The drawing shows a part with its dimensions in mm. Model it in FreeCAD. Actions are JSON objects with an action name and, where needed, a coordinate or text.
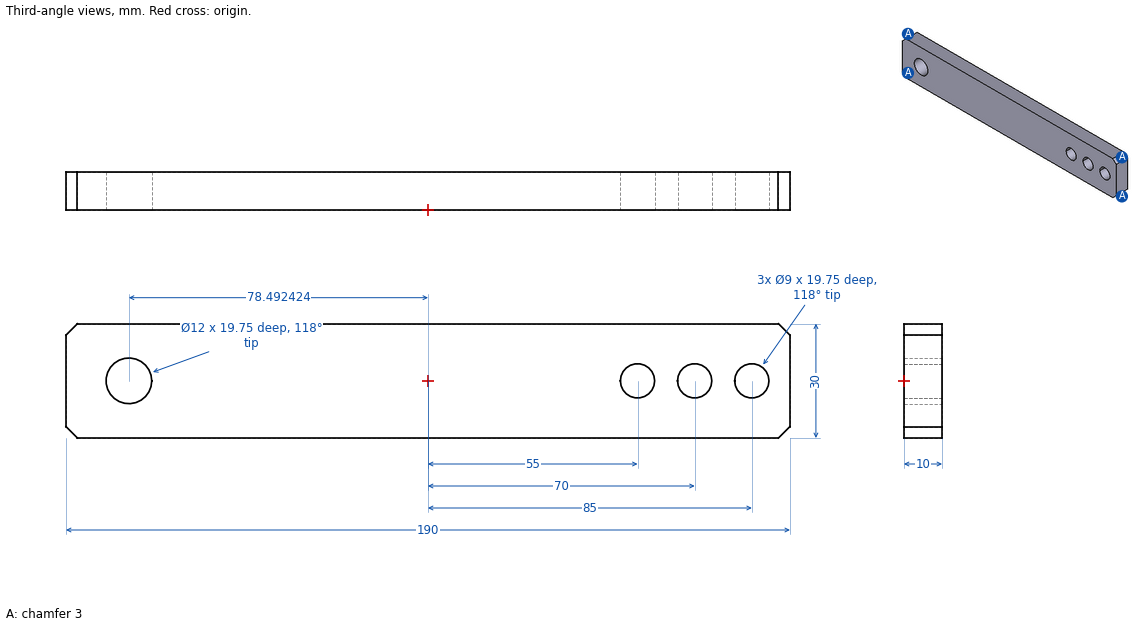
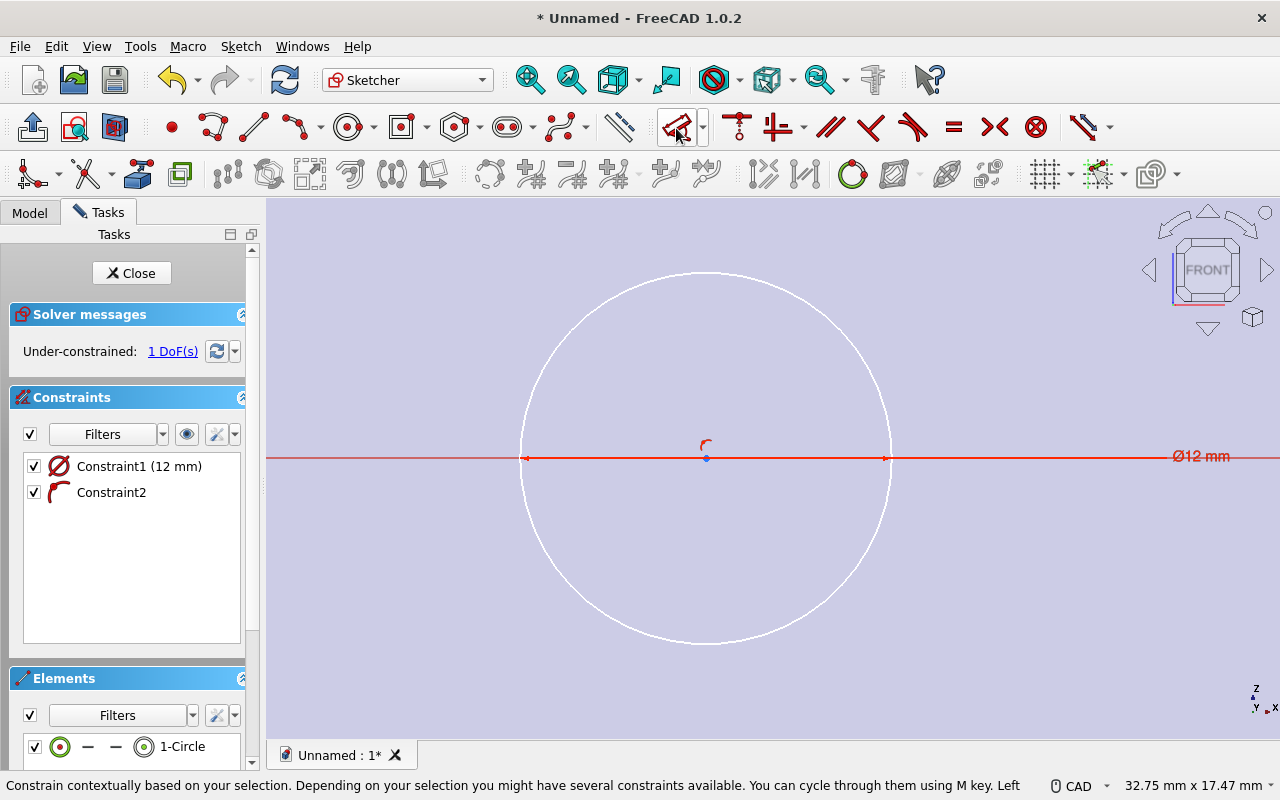
{"action": "left_click", "coordinate": [706, 458]}
{"action": "left_click", "coordinate": [911, 492]}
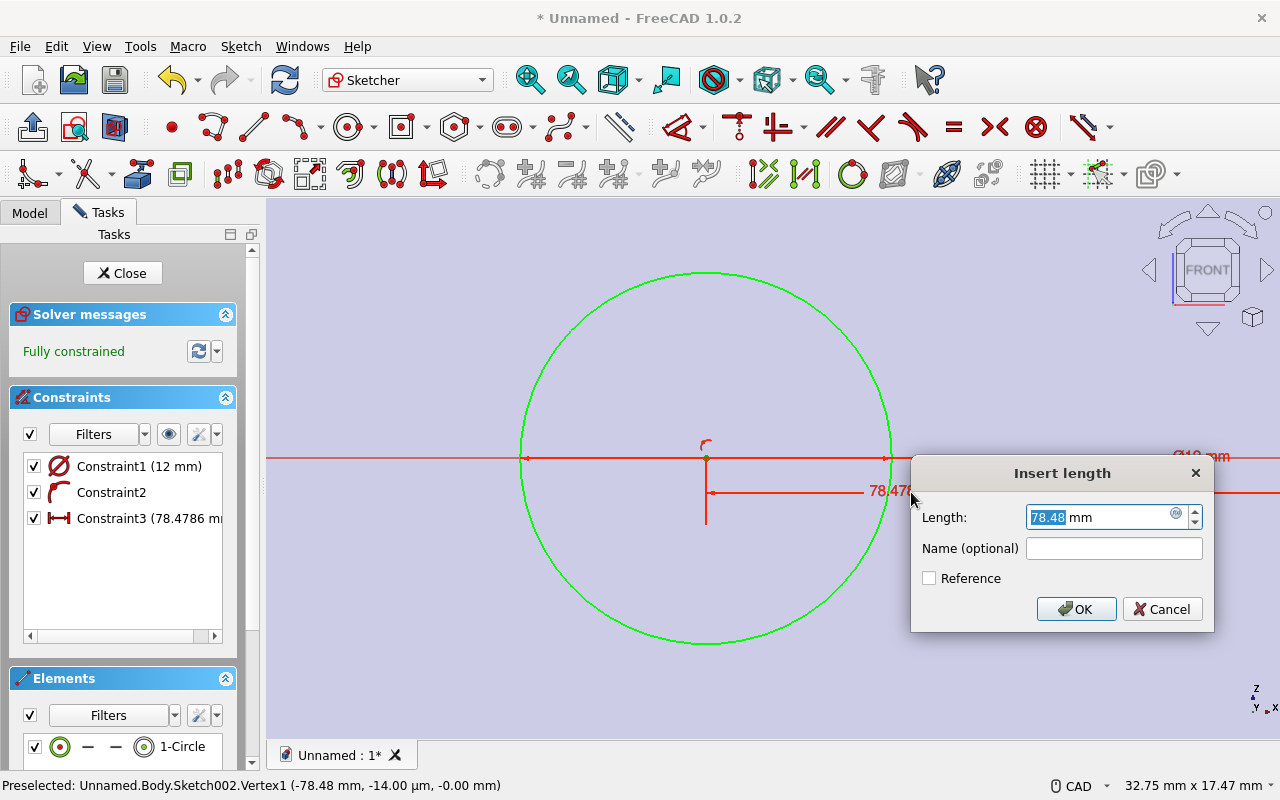
{"action": "type", "text": "78.492424"}
{"action": "key", "text": "Return"}
{"action": "key", "text": "Escape"}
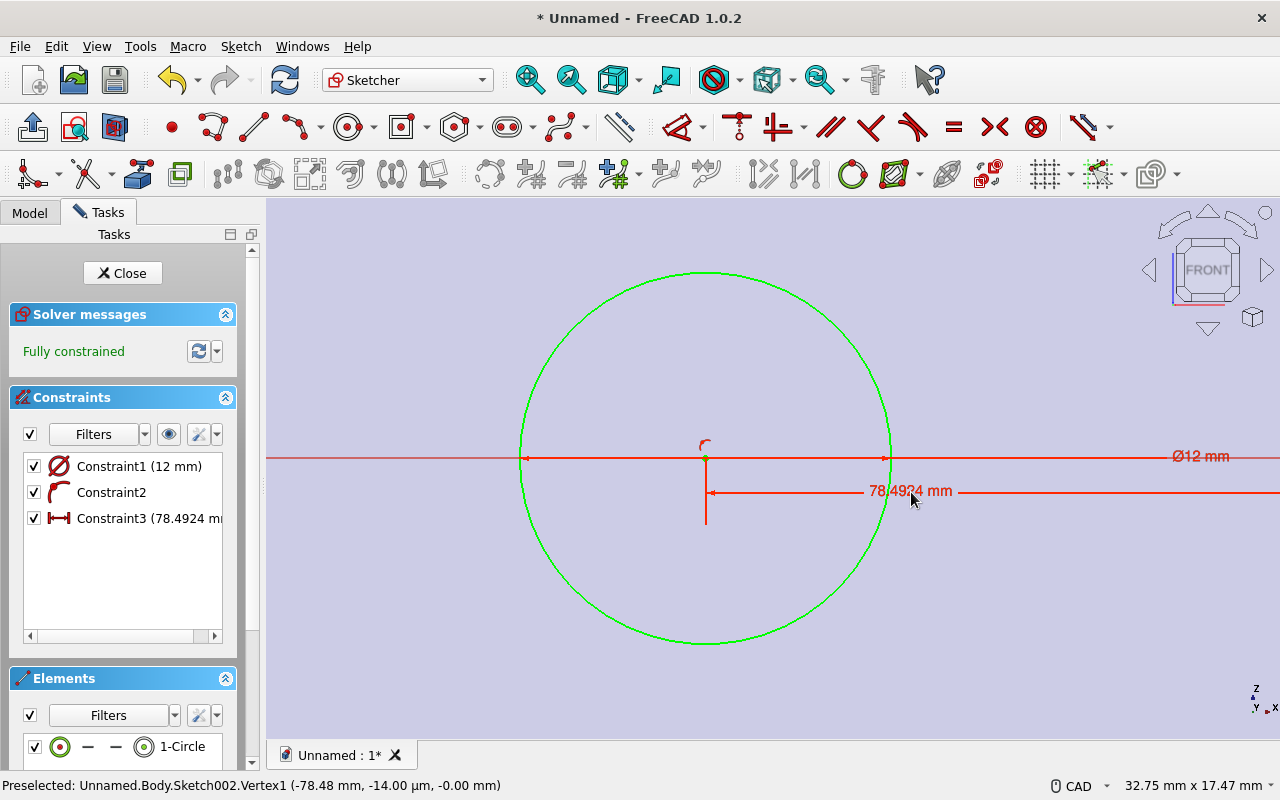
{"action": "left_click", "coordinate": [123, 273]}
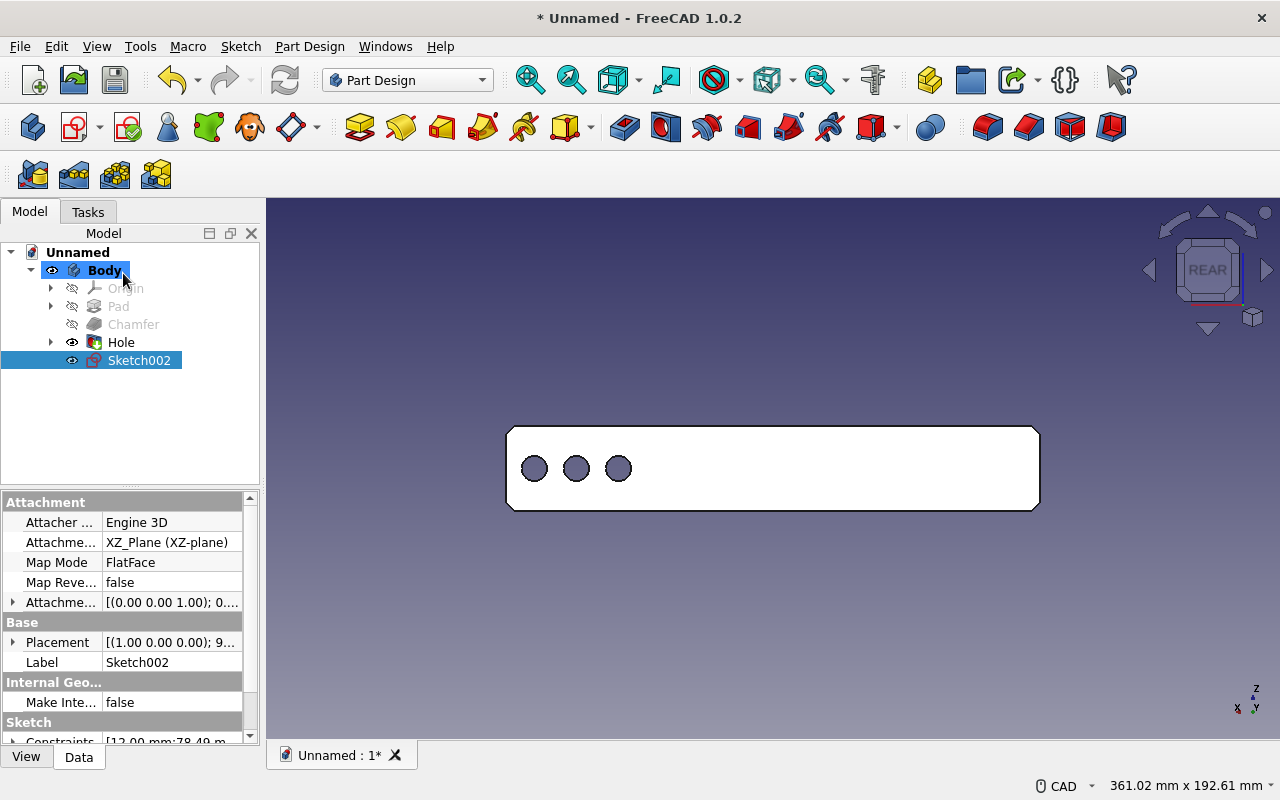
{"action": "left_click", "coordinate": [666, 128]}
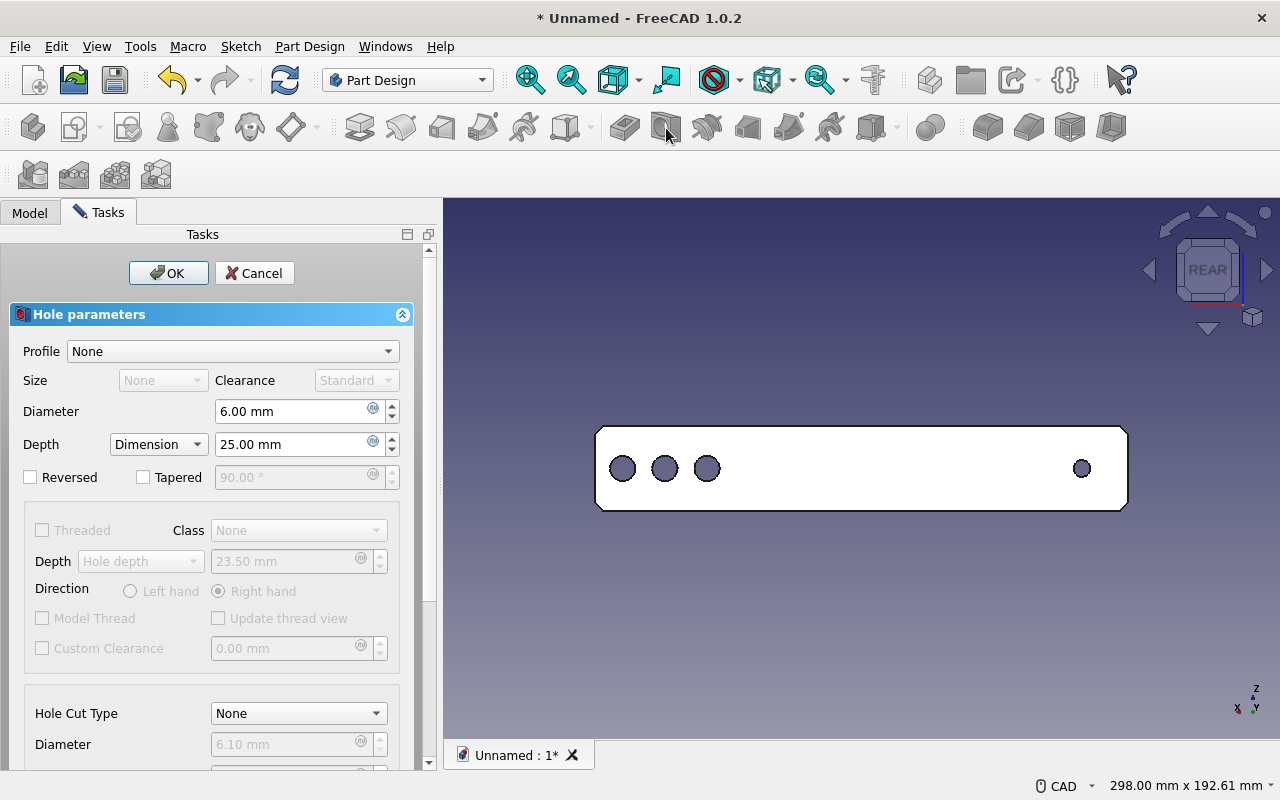
{"action": "triple_click", "coordinate": [300, 412]}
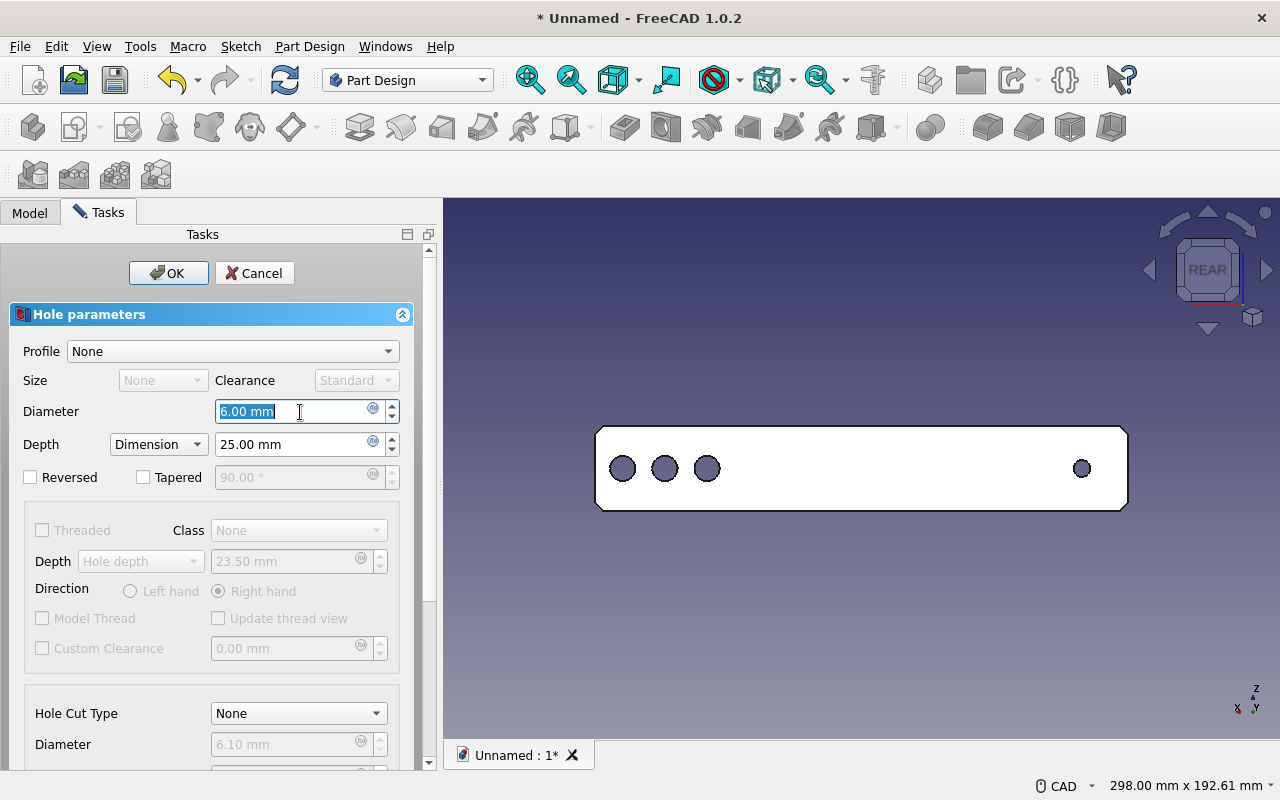
{"action": "type", "text": "12"}
{"action": "key", "text": "Tab"}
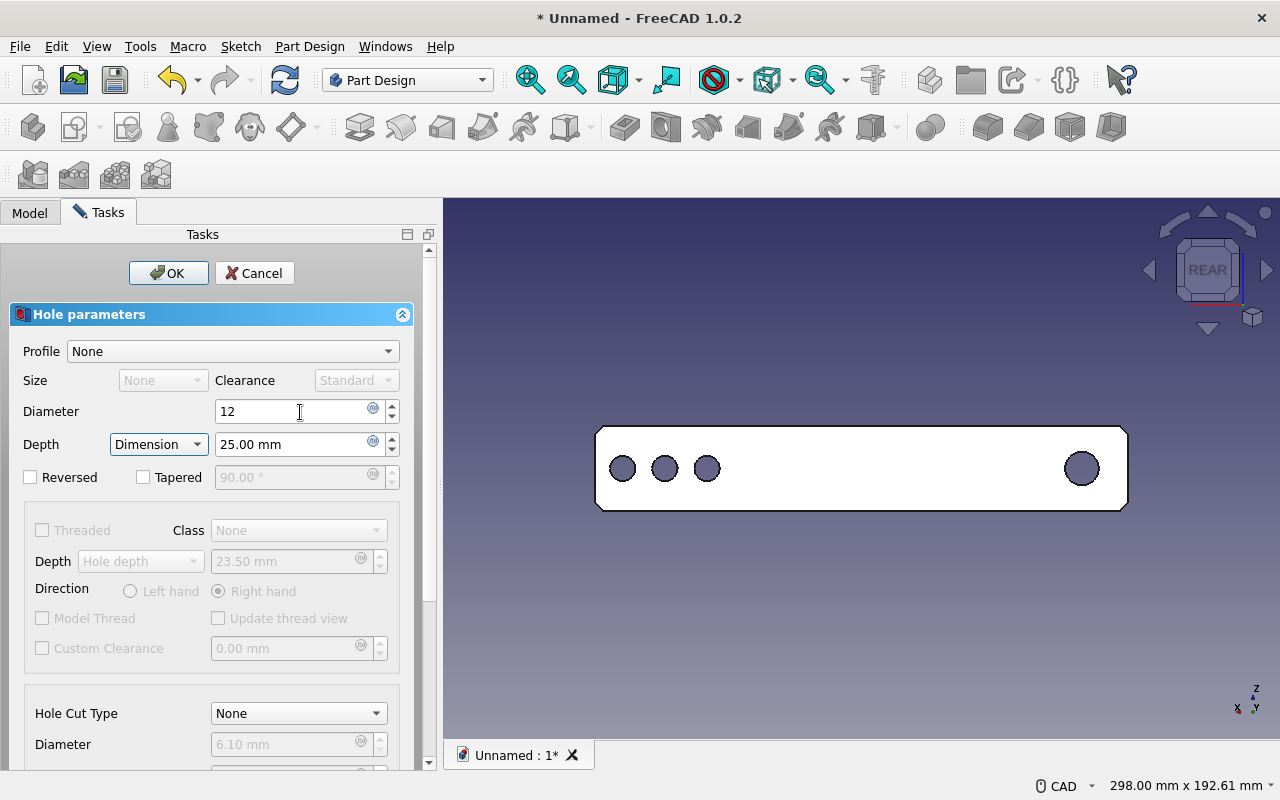
{"action": "triple_click", "coordinate": [300, 444]}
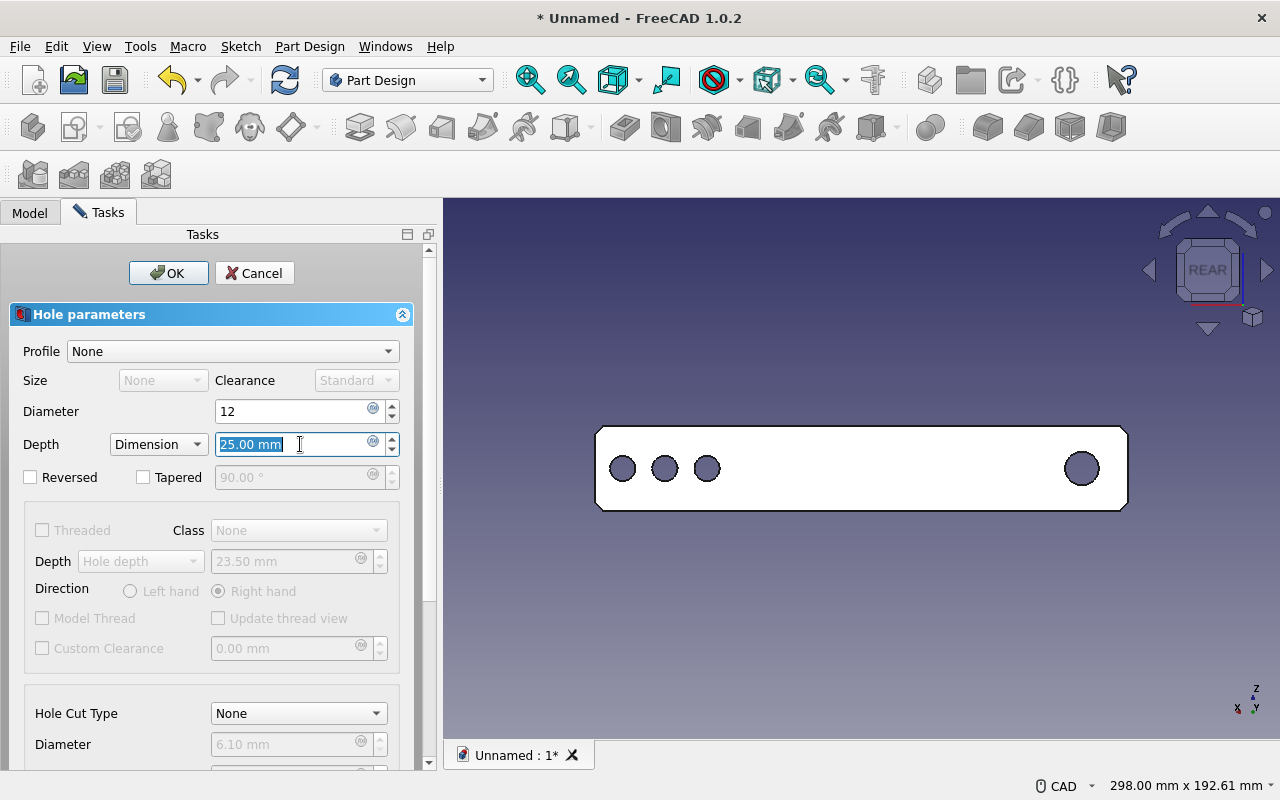
{"action": "type", "text": "19.75"}
{"action": "key", "text": "Tab"}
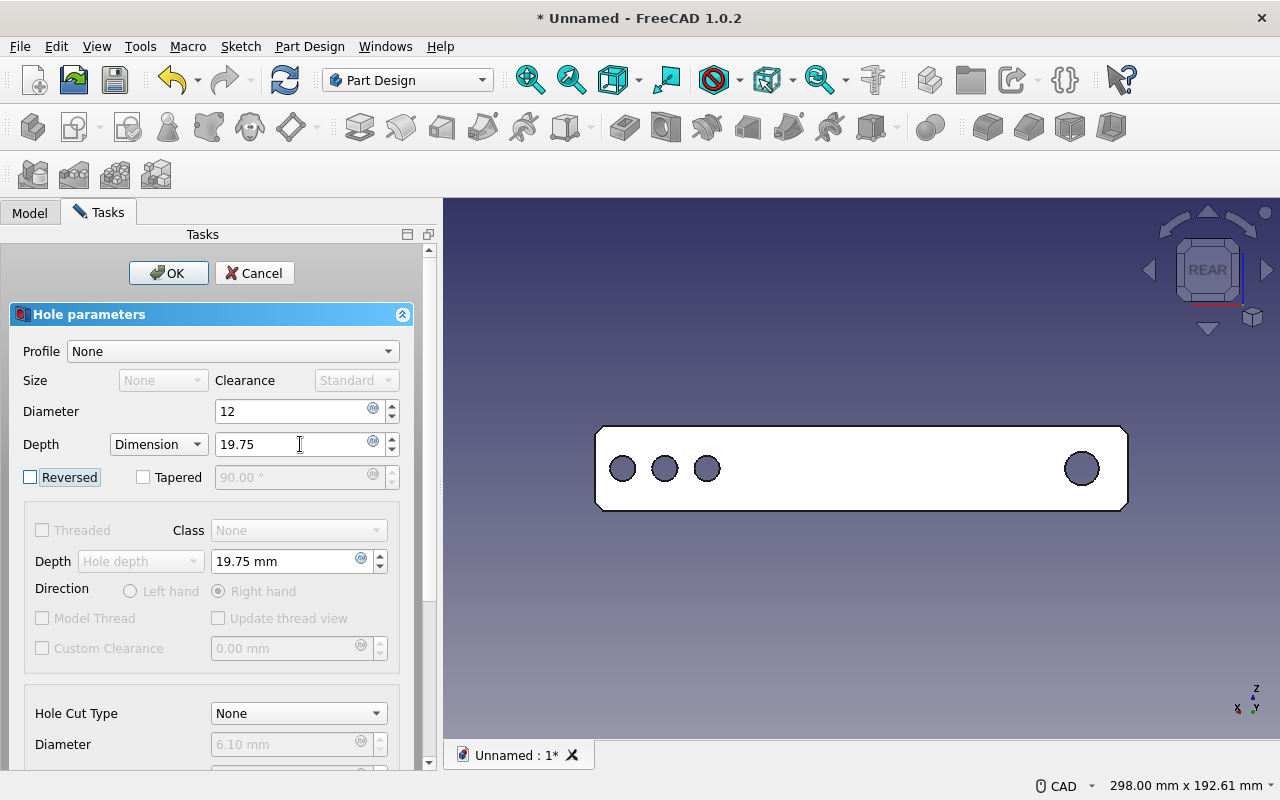
{"action": "left_click", "coordinate": [169, 273]}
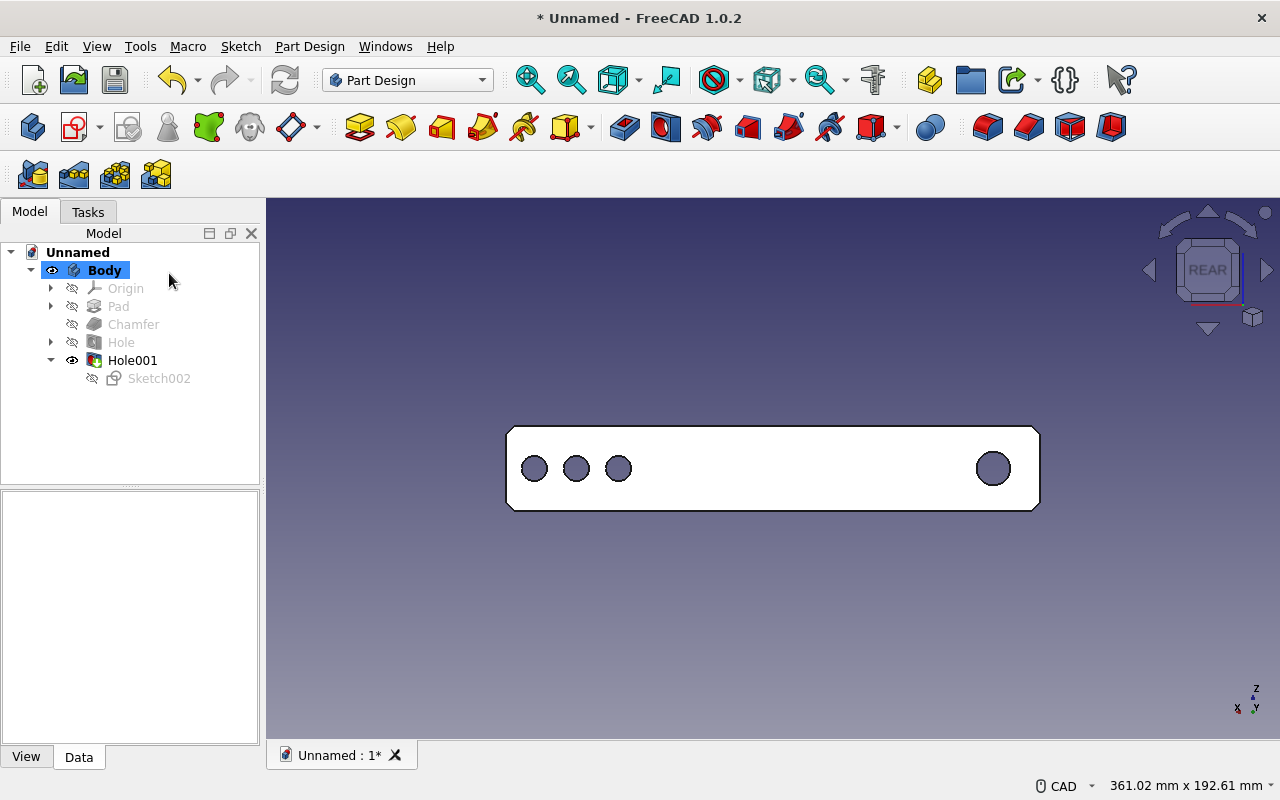
{"action": "key", "text": "0"}